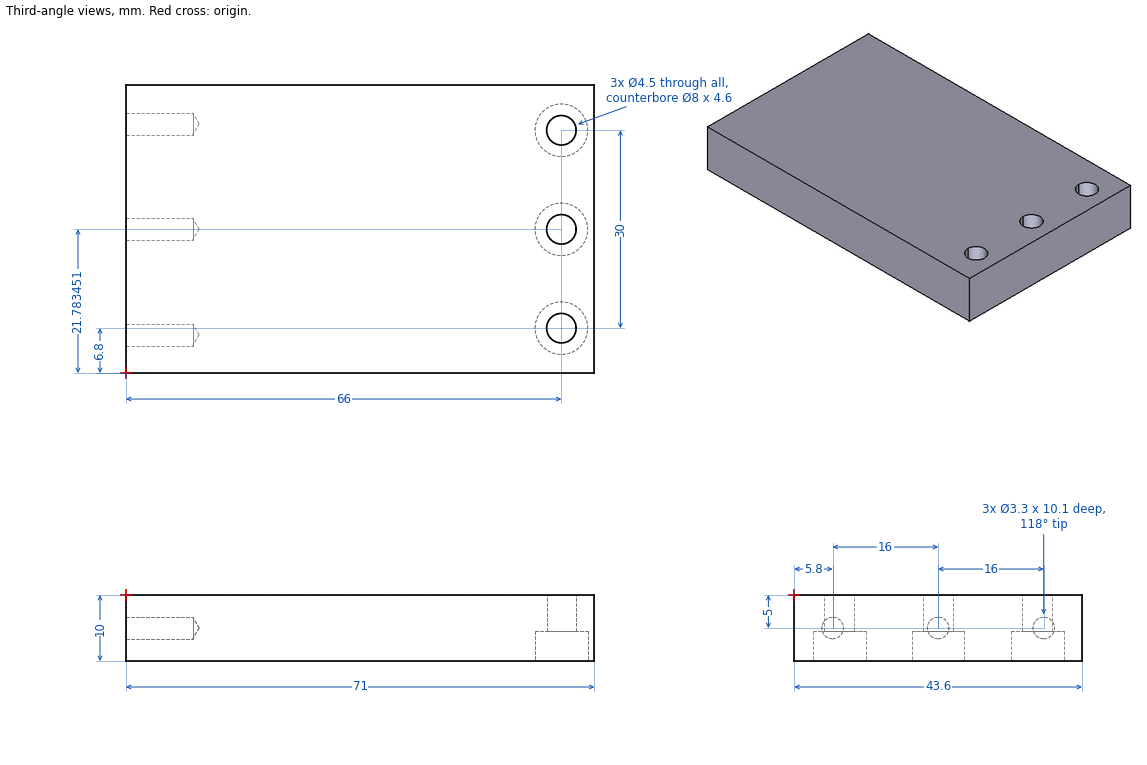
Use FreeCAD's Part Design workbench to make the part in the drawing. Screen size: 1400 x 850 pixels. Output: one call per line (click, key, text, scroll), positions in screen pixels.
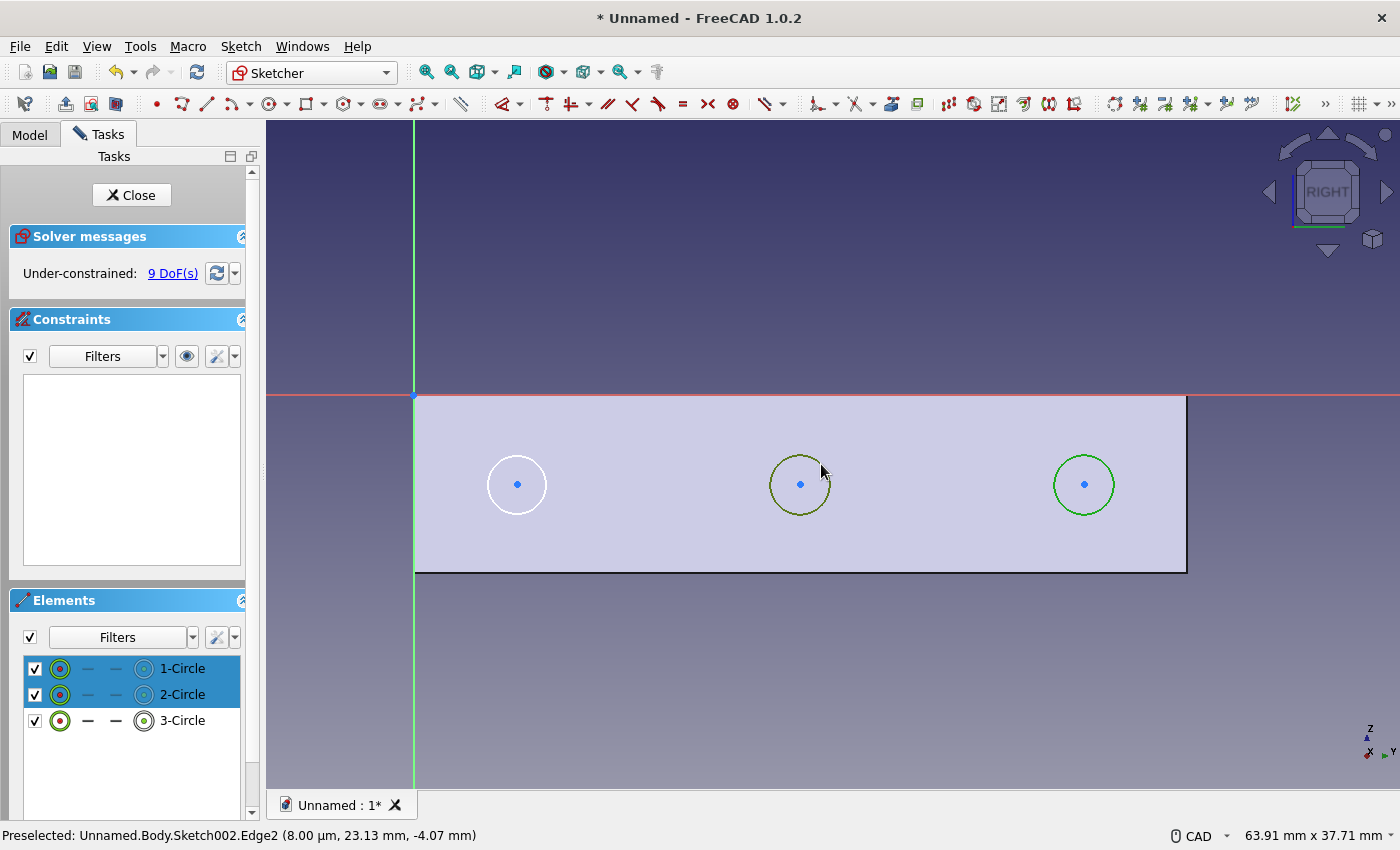
click(537, 464)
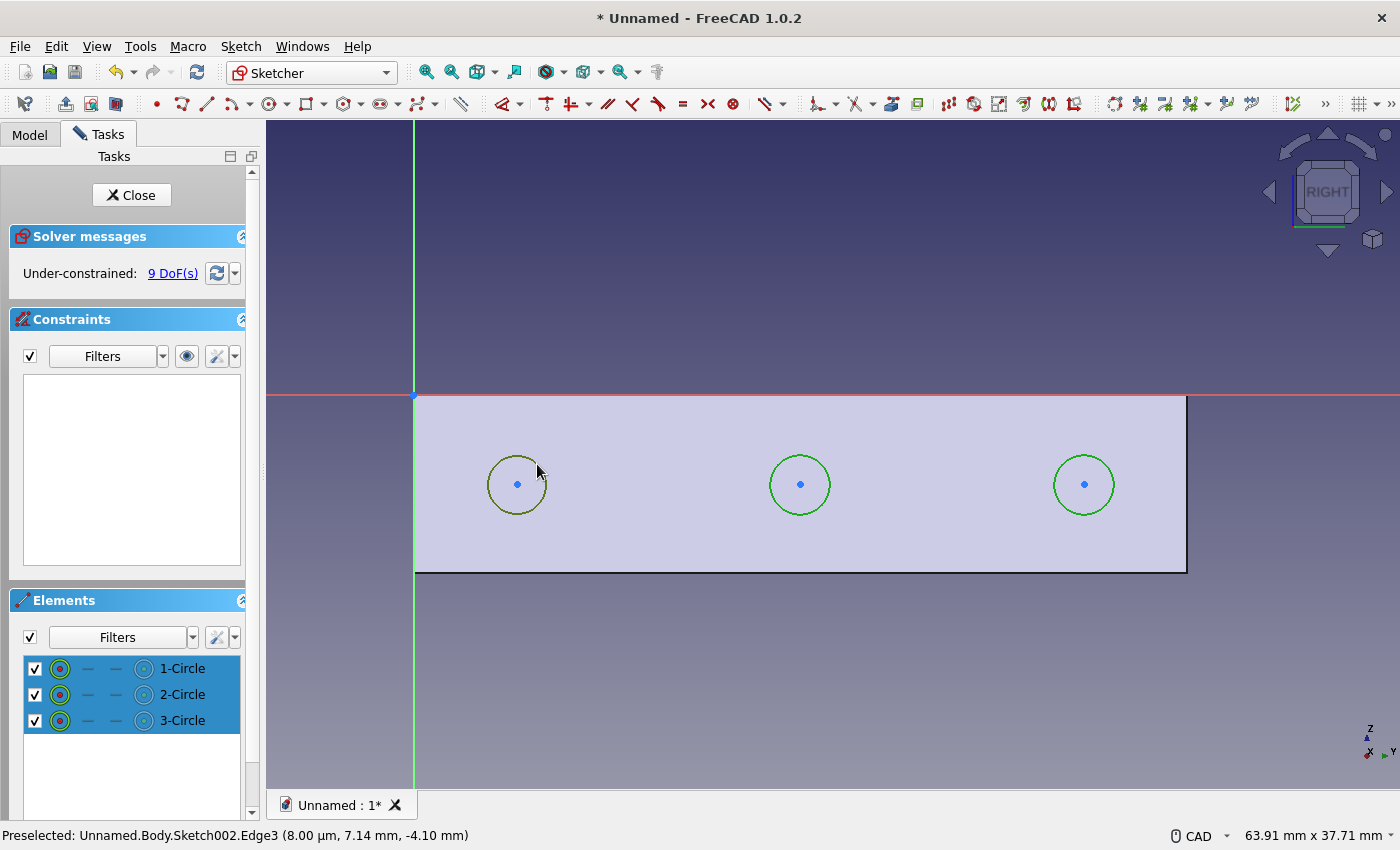
key(e)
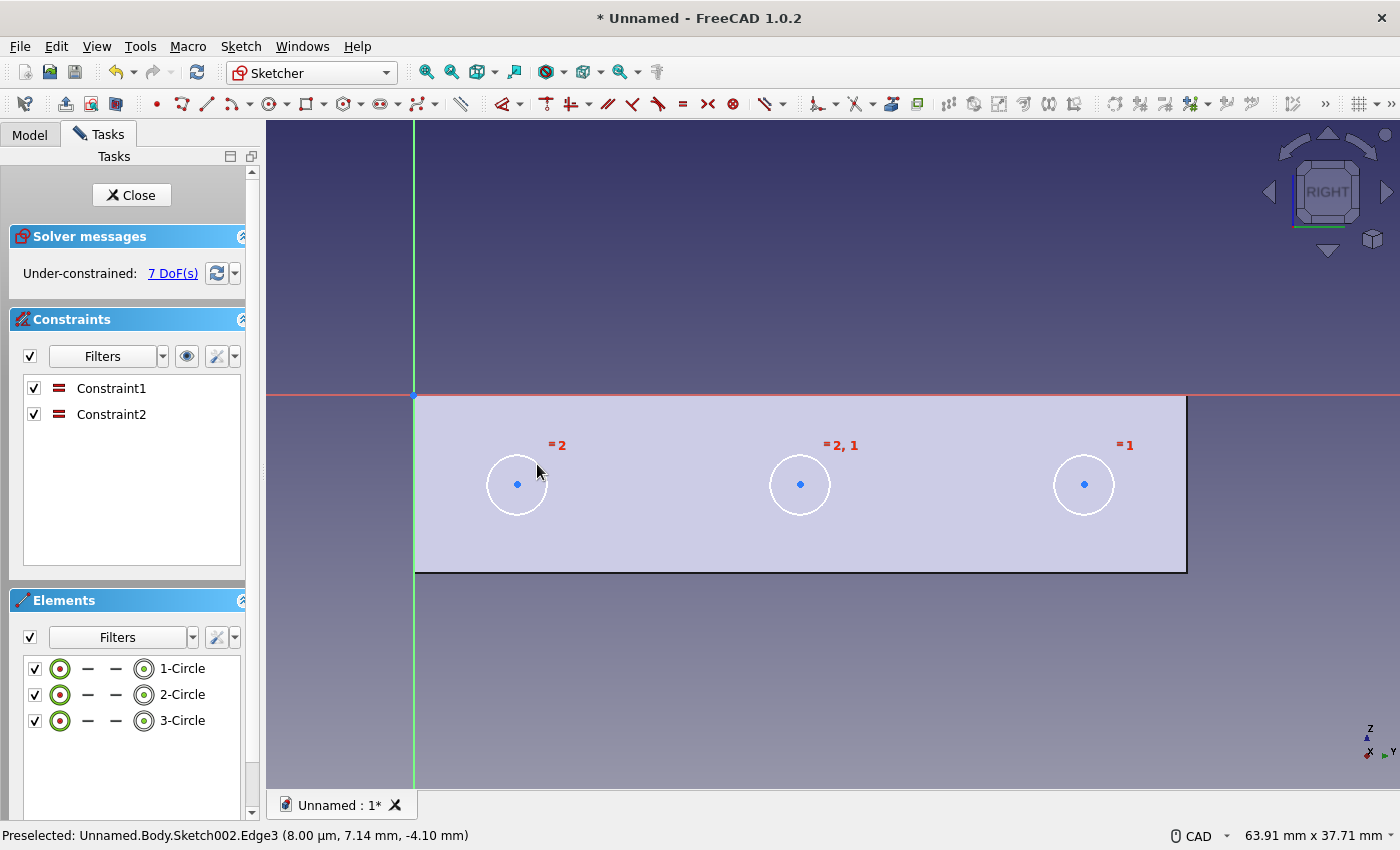
click(1084, 485)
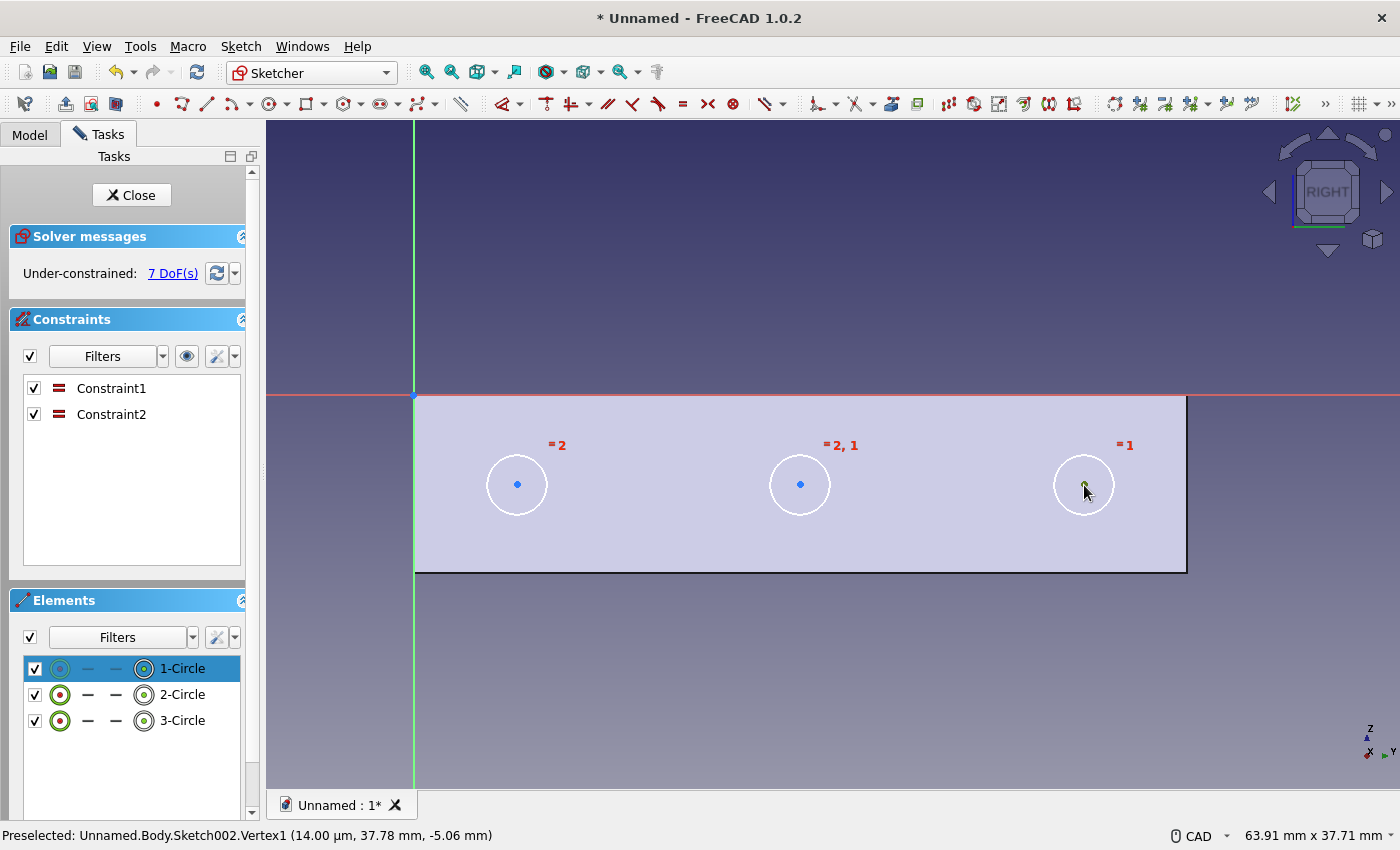
click(800, 485)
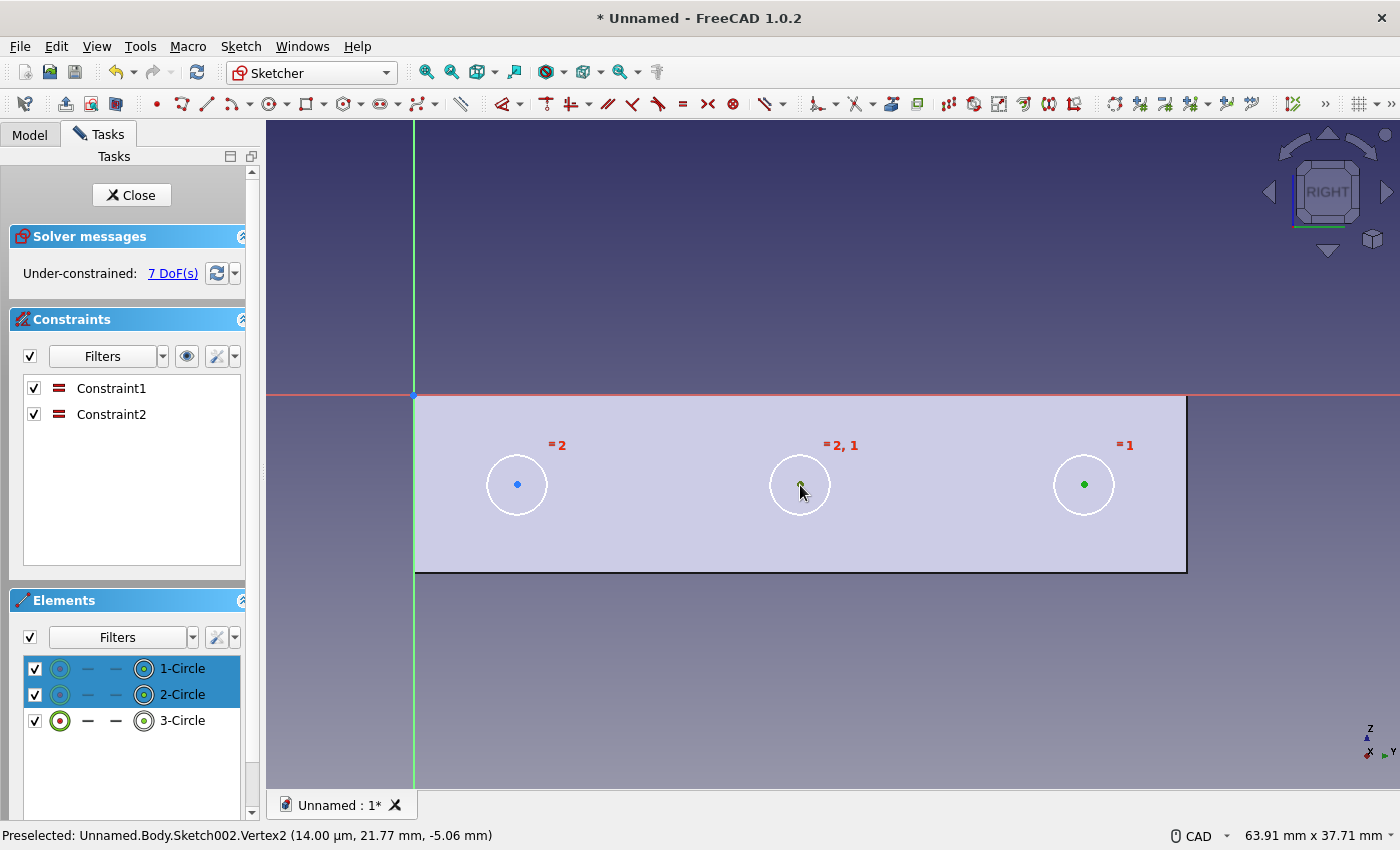
key(h)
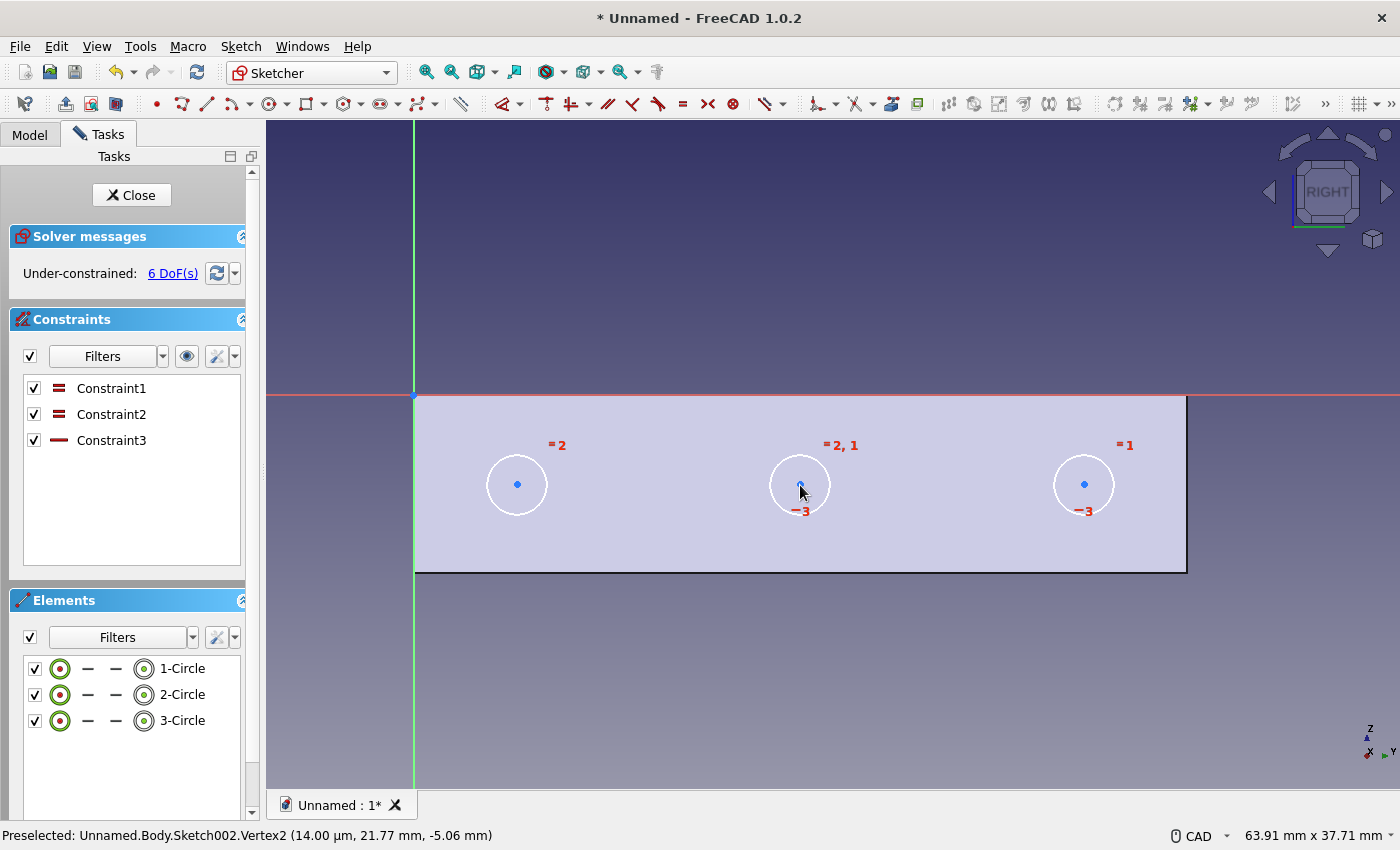
click(800, 485)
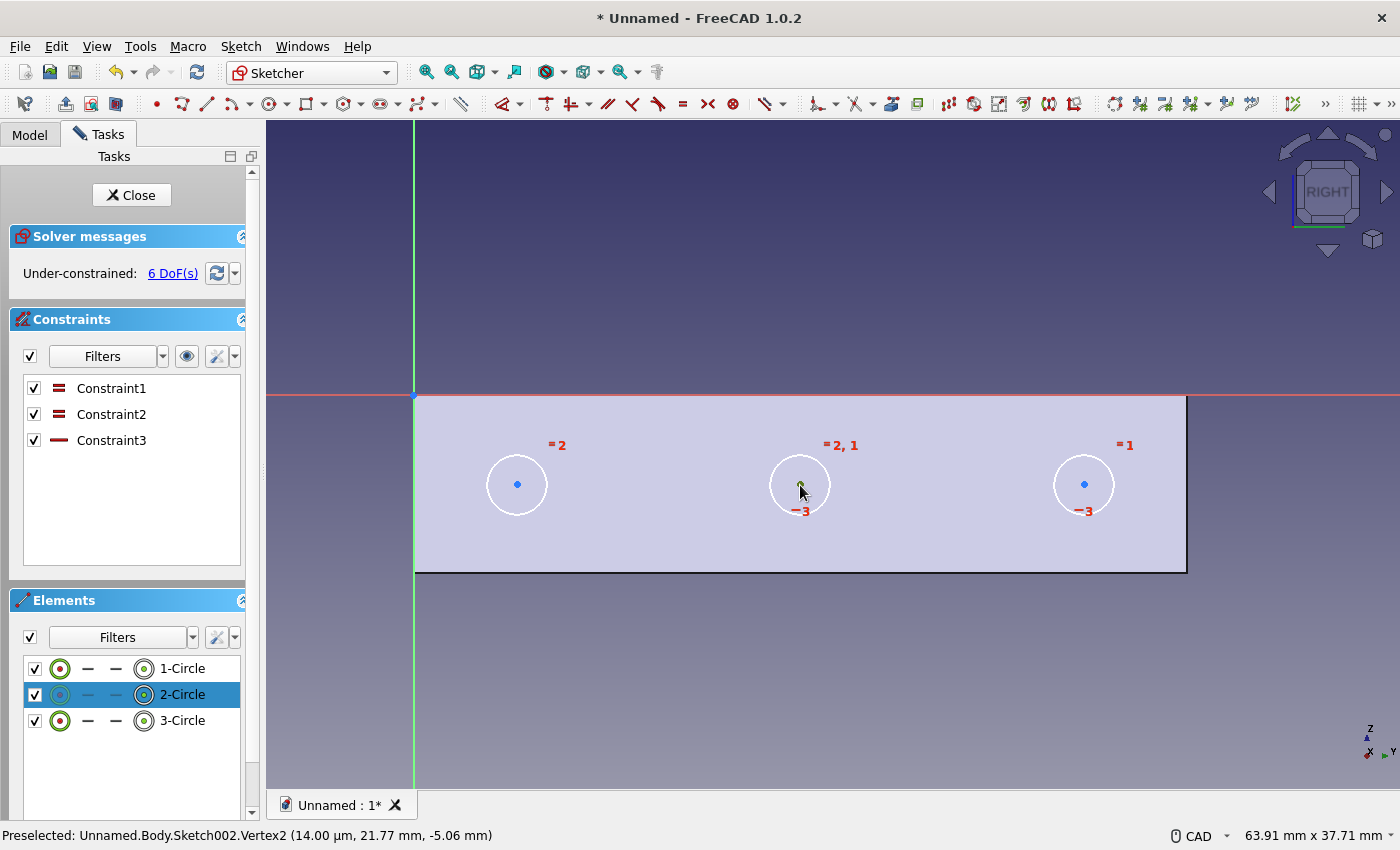
click(517, 485)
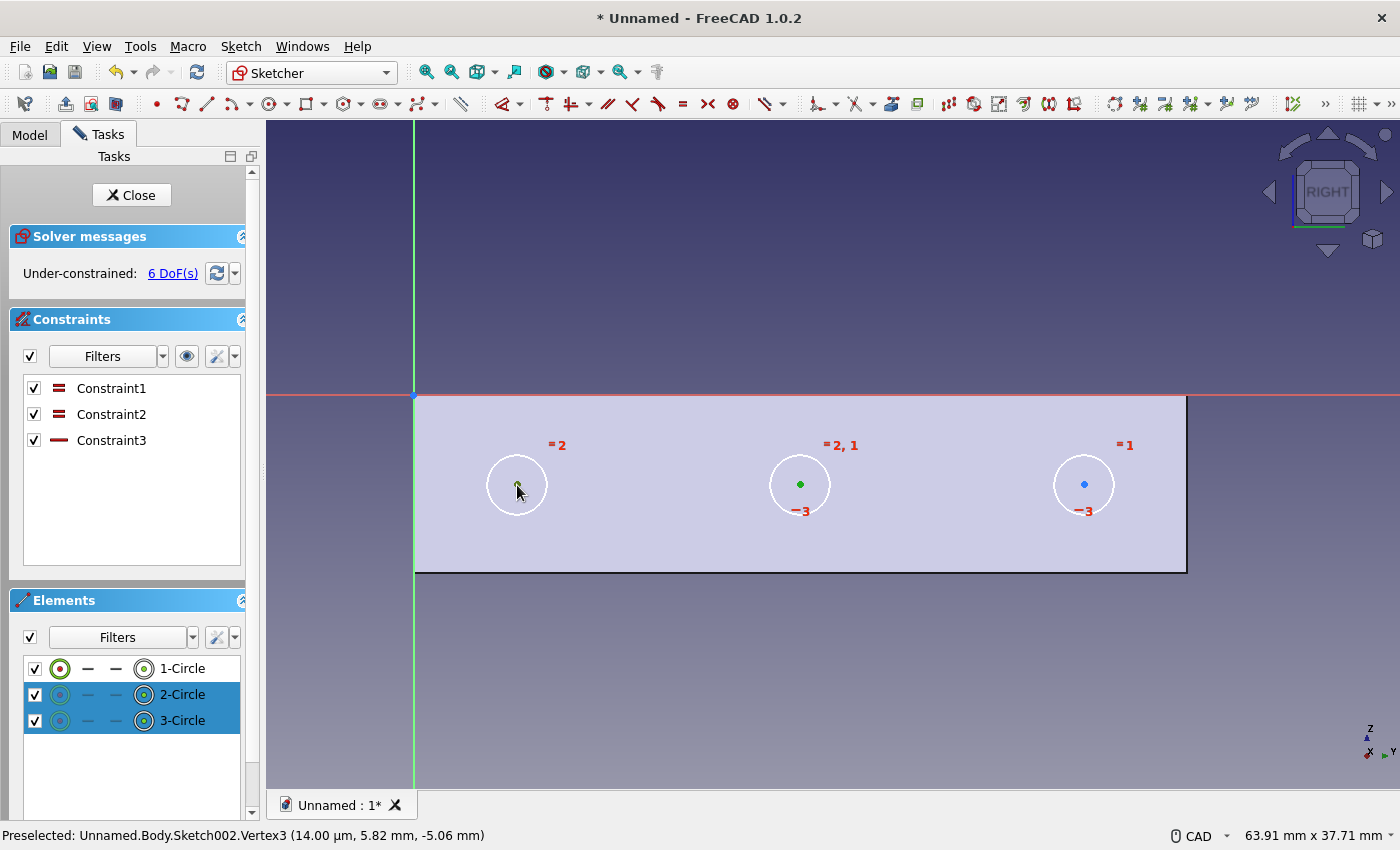
key(h)